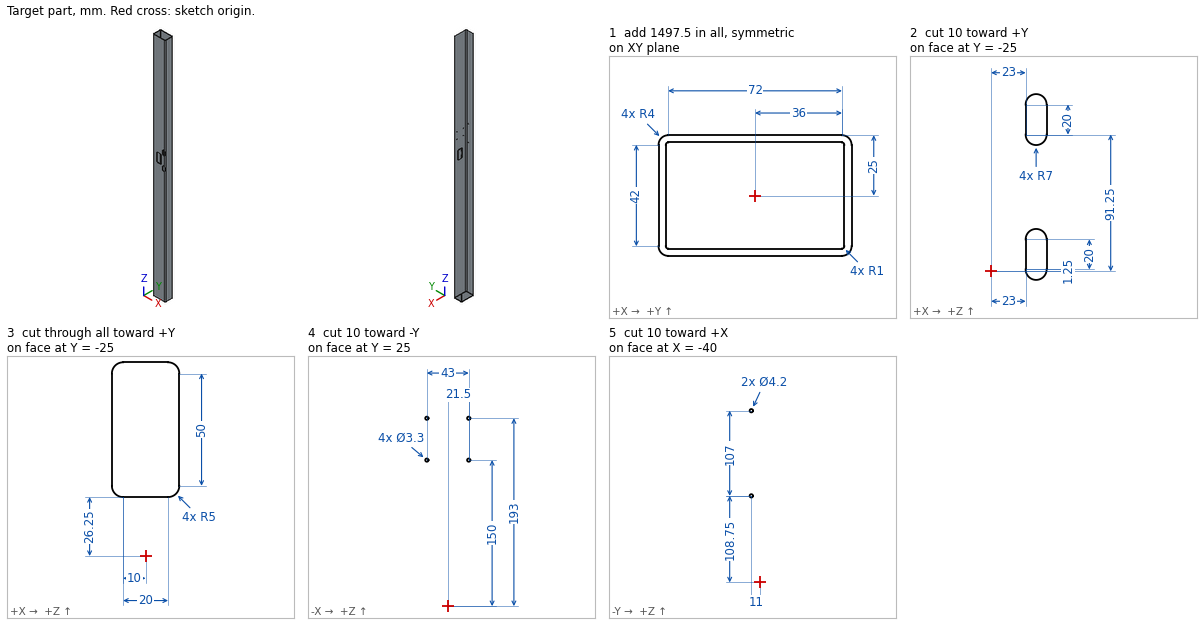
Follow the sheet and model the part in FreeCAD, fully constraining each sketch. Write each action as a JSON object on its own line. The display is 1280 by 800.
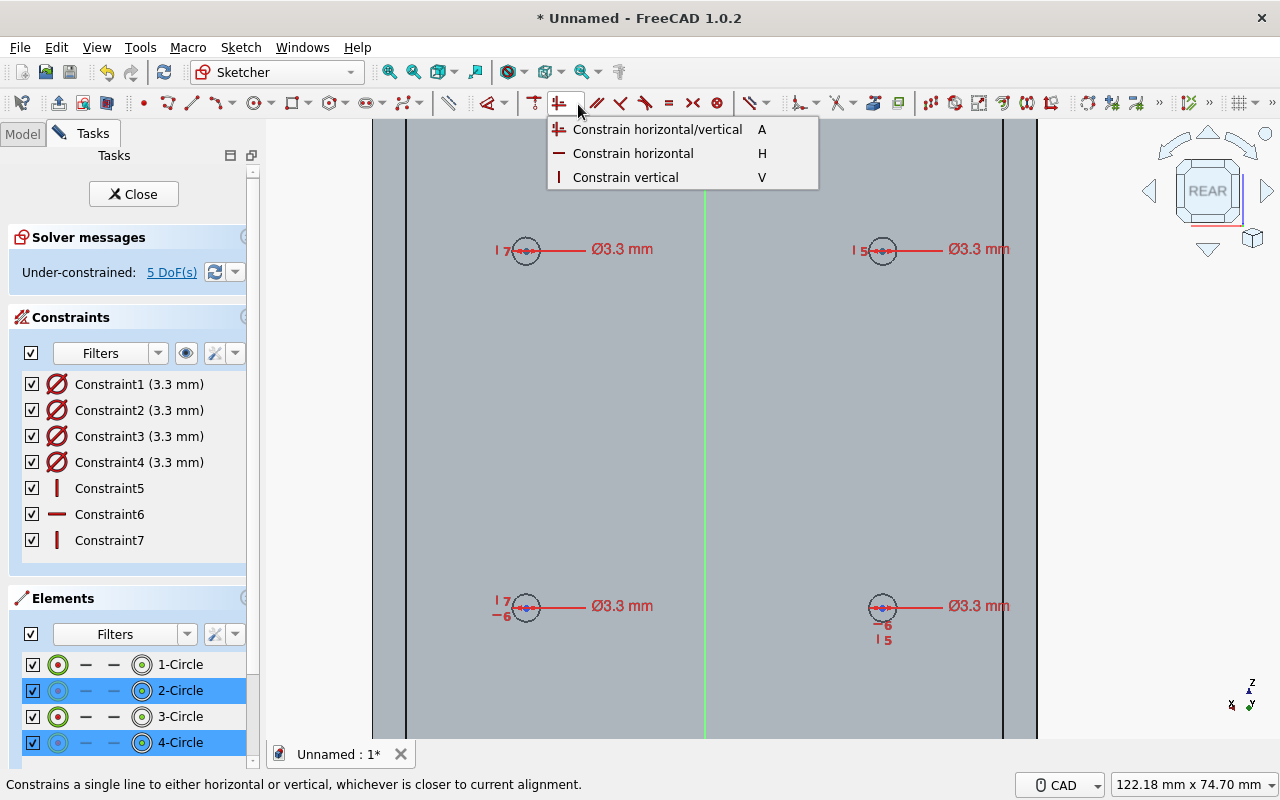
{"action": "left_click", "coordinate": [683, 153]}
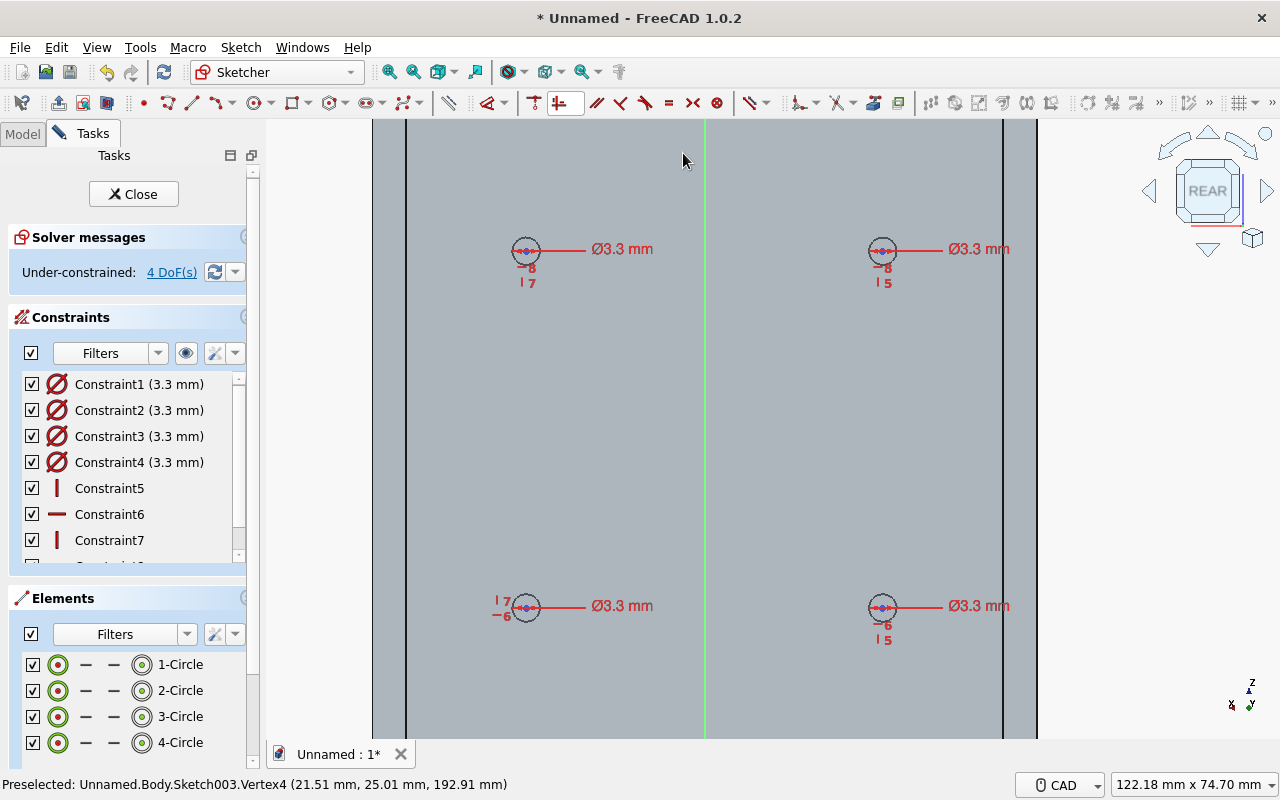
{"action": "left_click", "coordinate": [488, 104]}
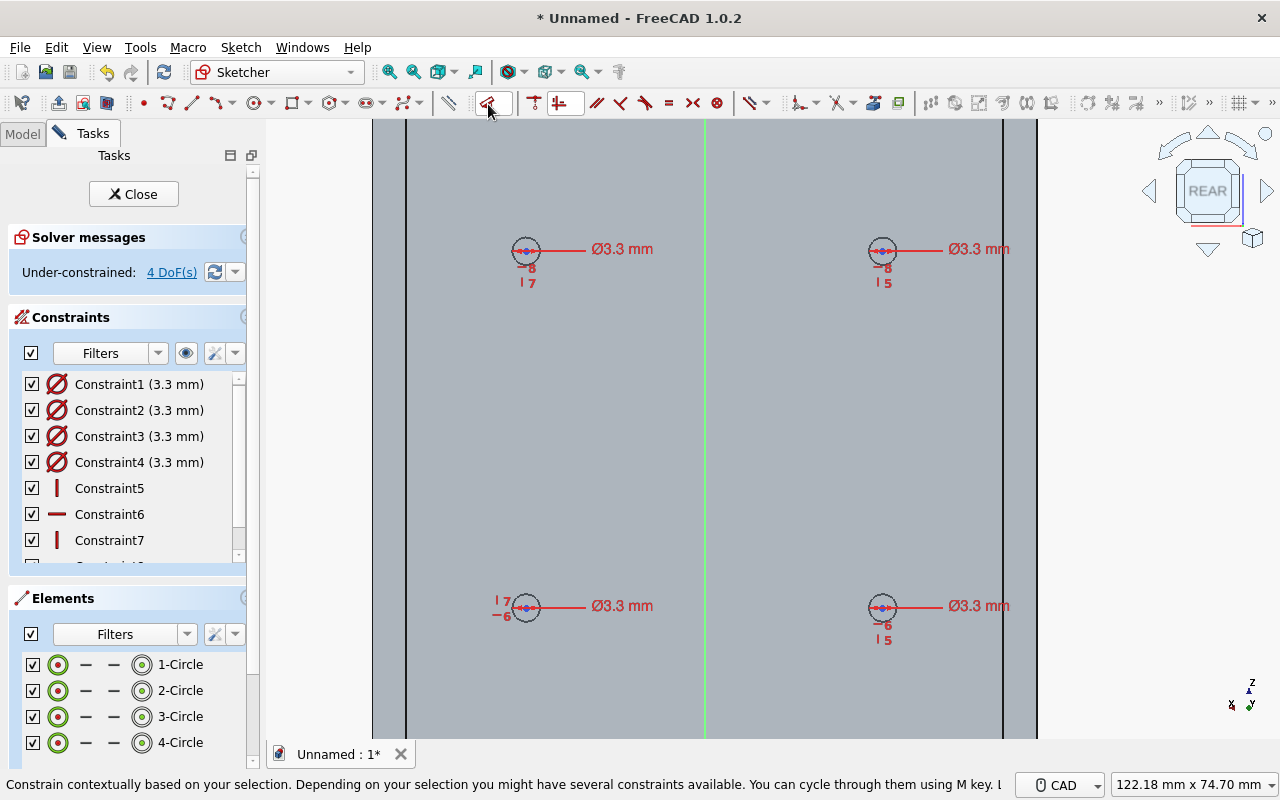
{"action": "left_click", "coordinate": [883, 608]}
{"action": "left_click", "coordinate": [917, 660]}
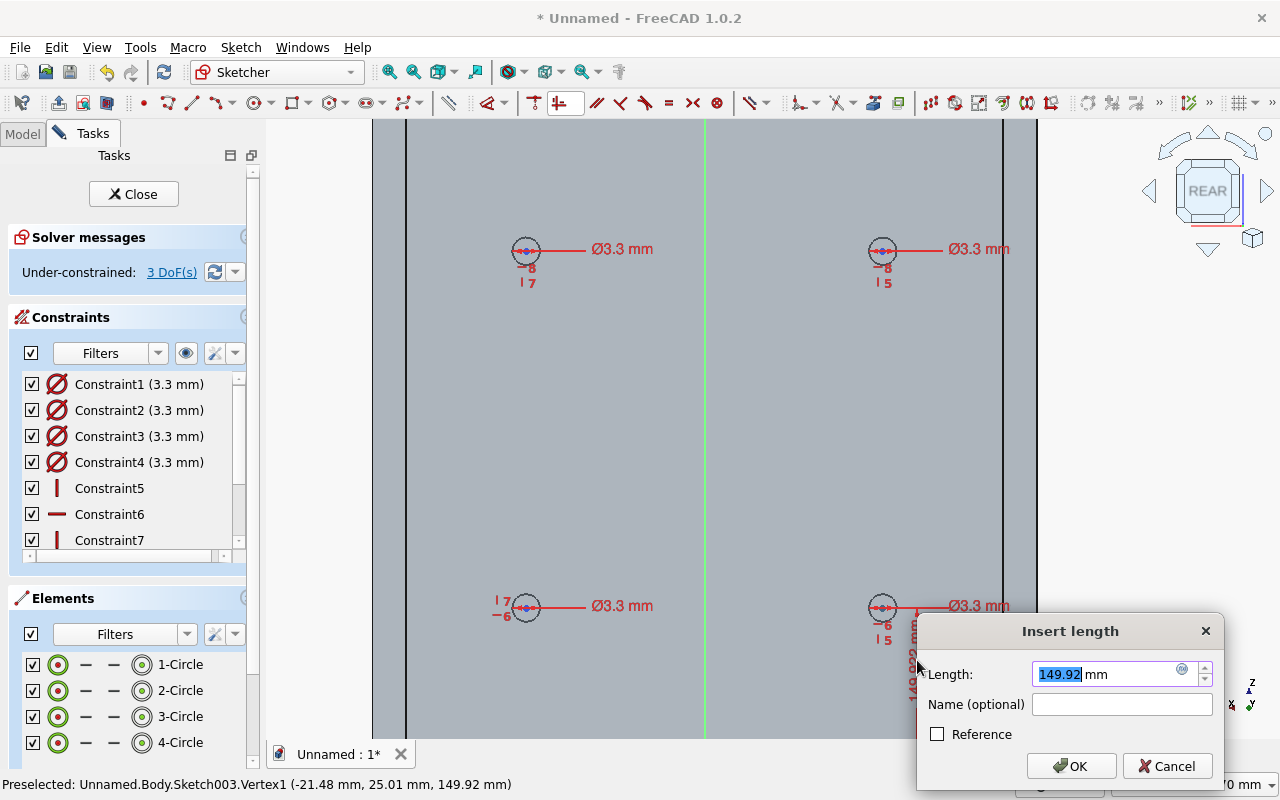
{"action": "type", "text": "150"}
{"action": "key", "text": "Return"}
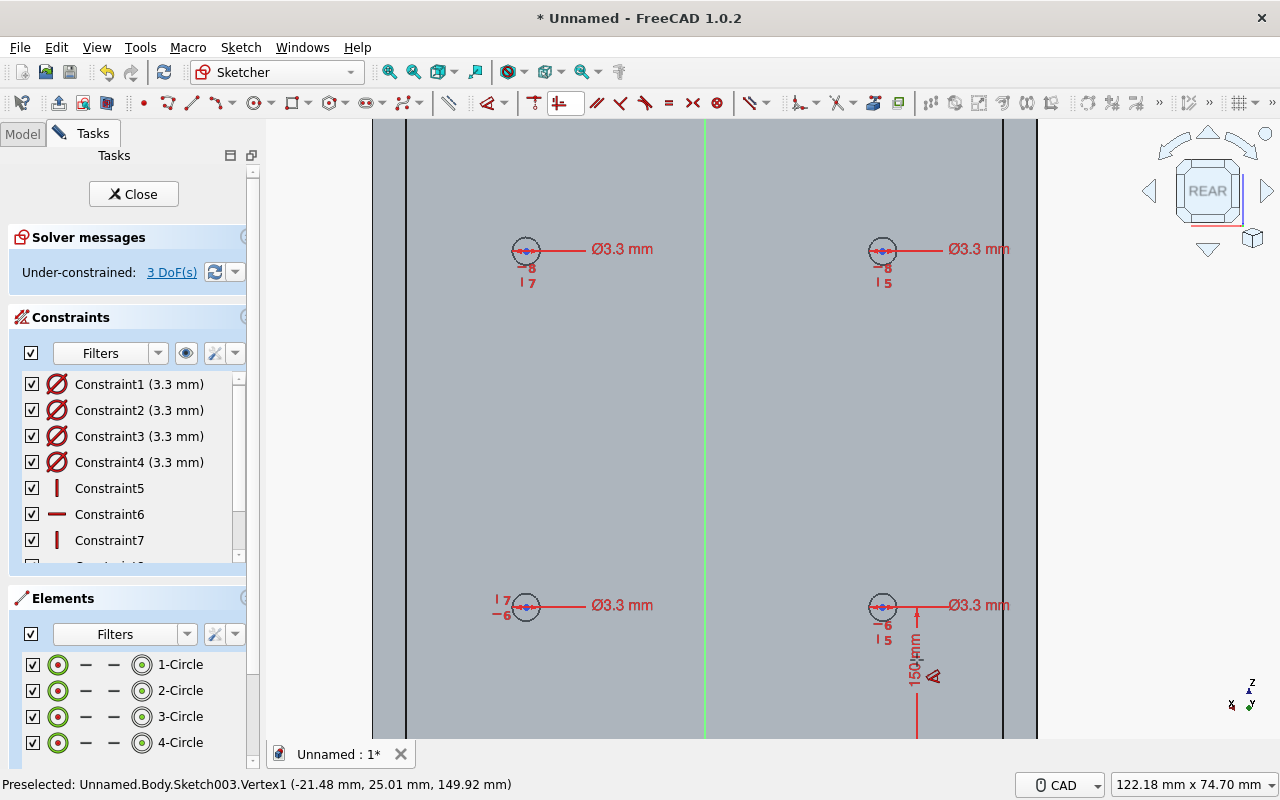
{"action": "left_click", "coordinate": [883, 251]}
{"action": "left_click", "coordinate": [917, 481]}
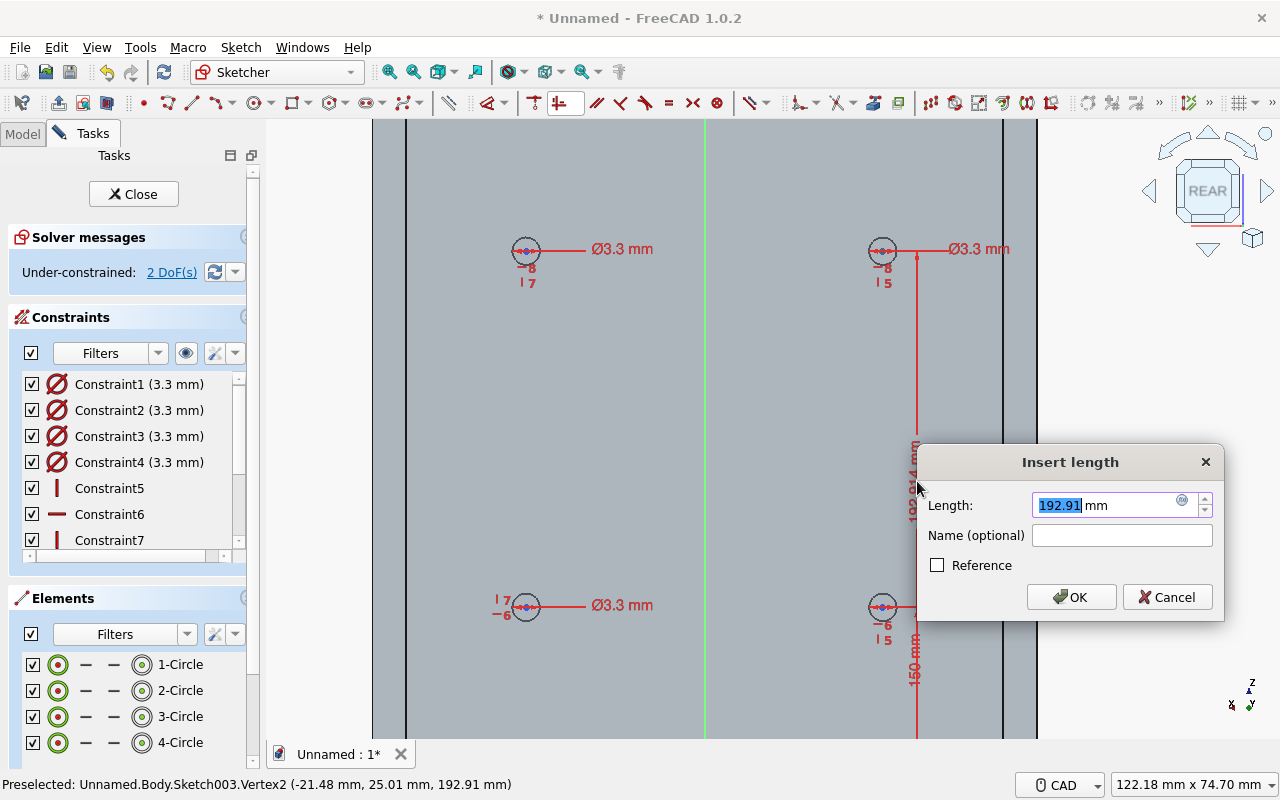
{"action": "type", "text": "193"}
{"action": "key", "text": "Return"}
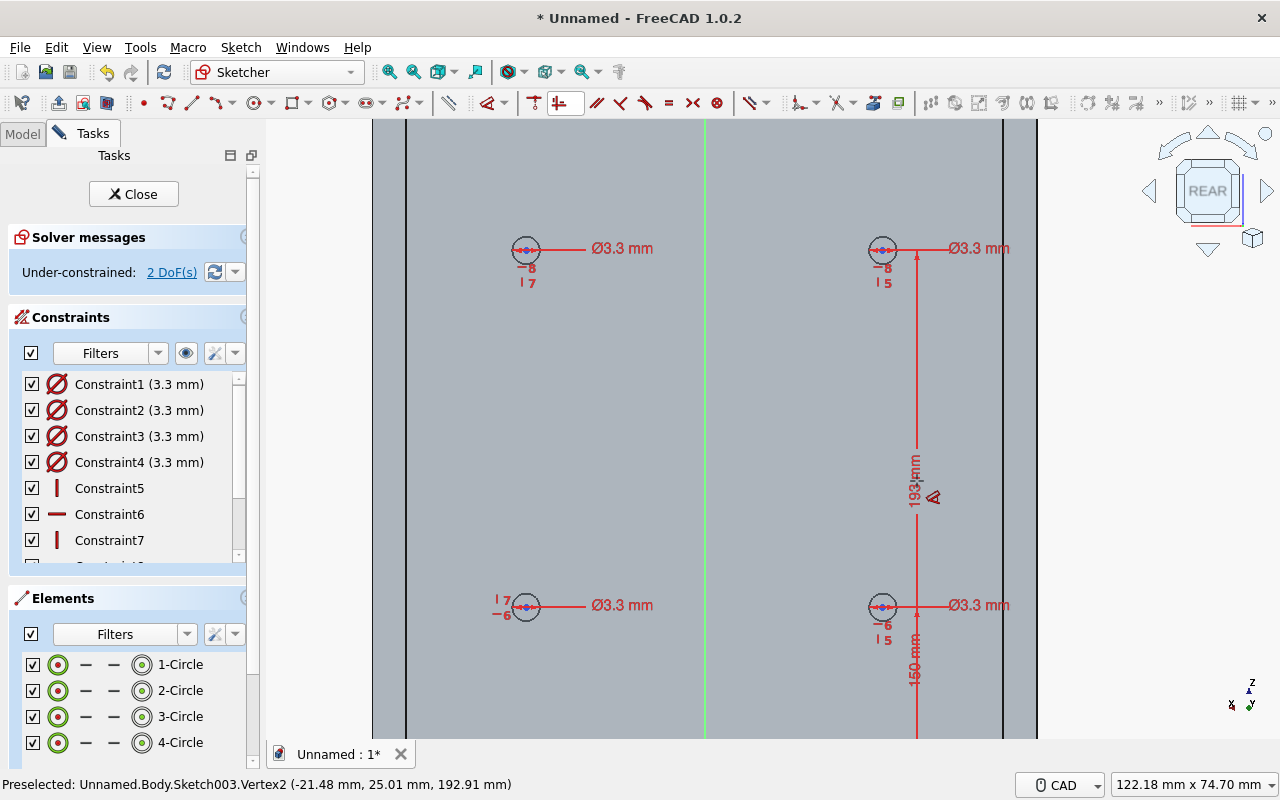
{"action": "left_click", "coordinate": [883, 607]}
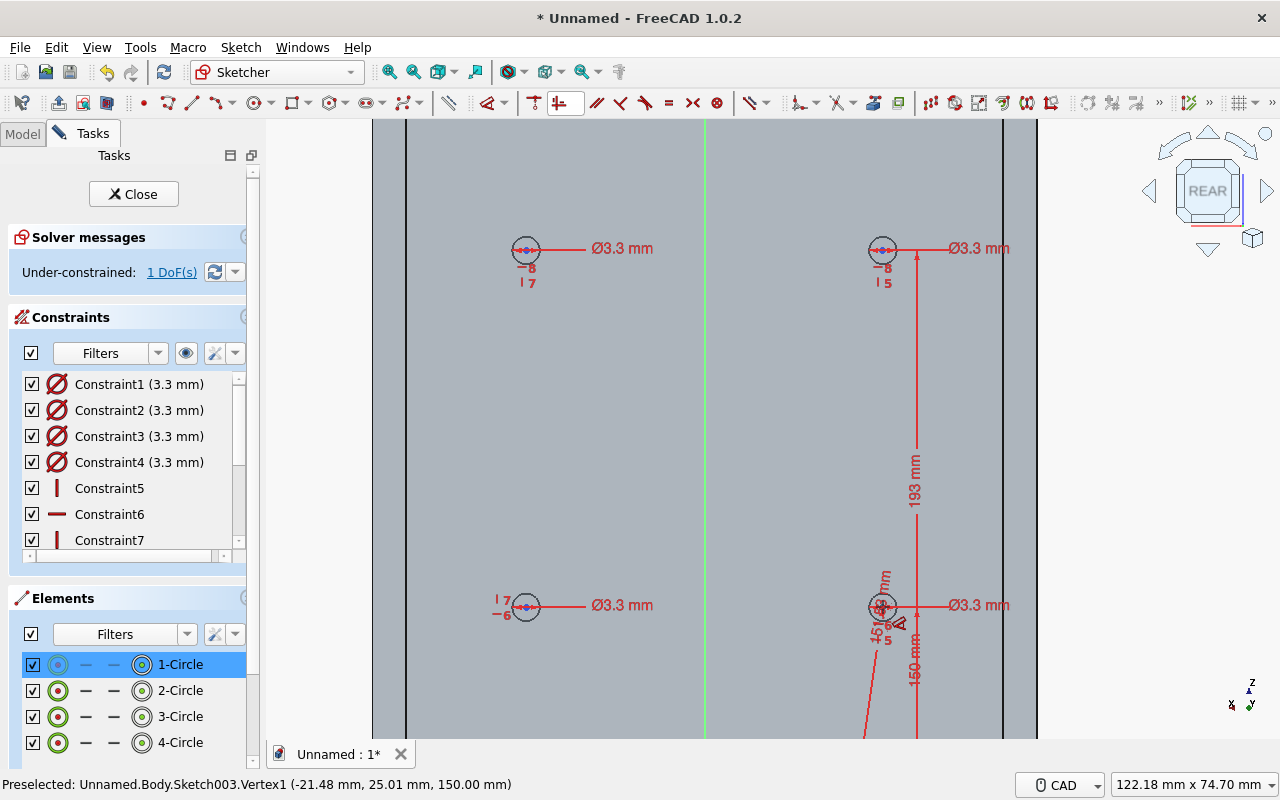
{"action": "left_click", "coordinate": [526, 607]}
{"action": "left_click", "coordinate": [622, 641]}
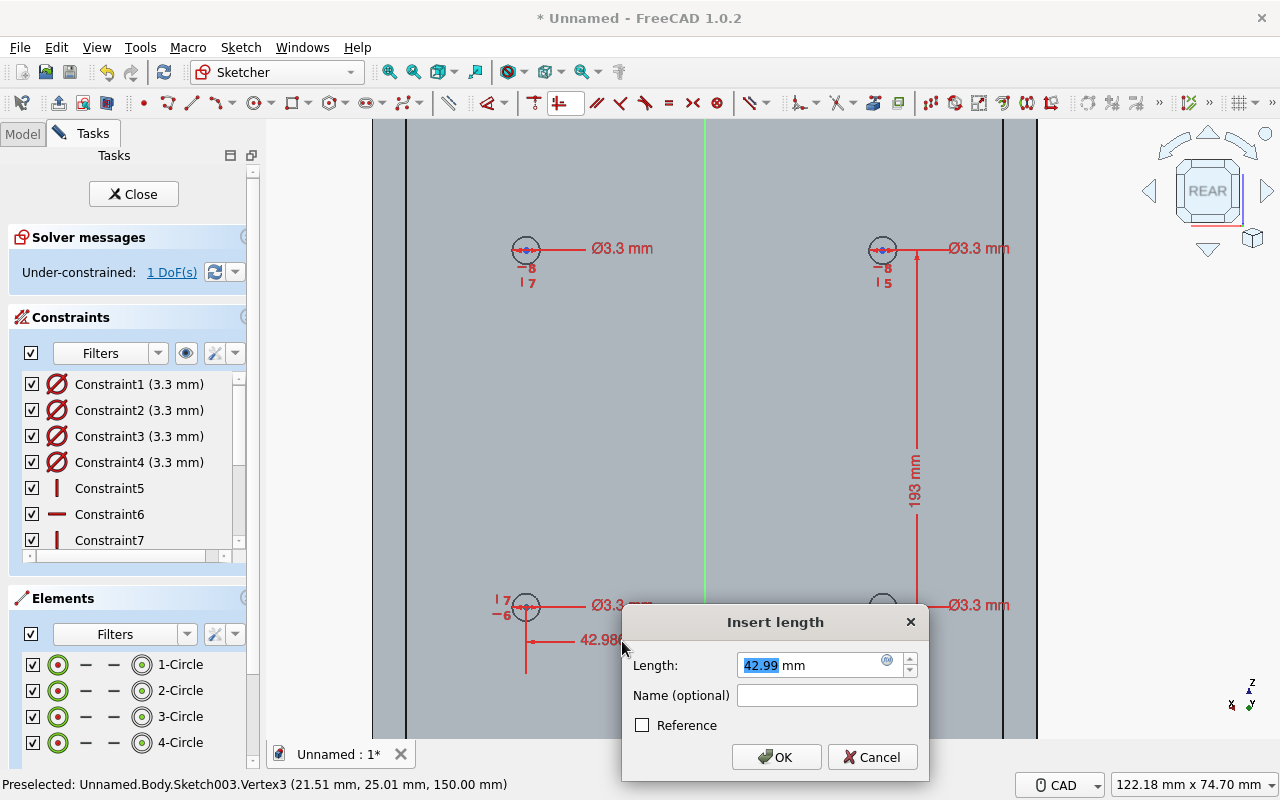
{"action": "type", "text": "43"}
{"action": "key", "text": "Return"}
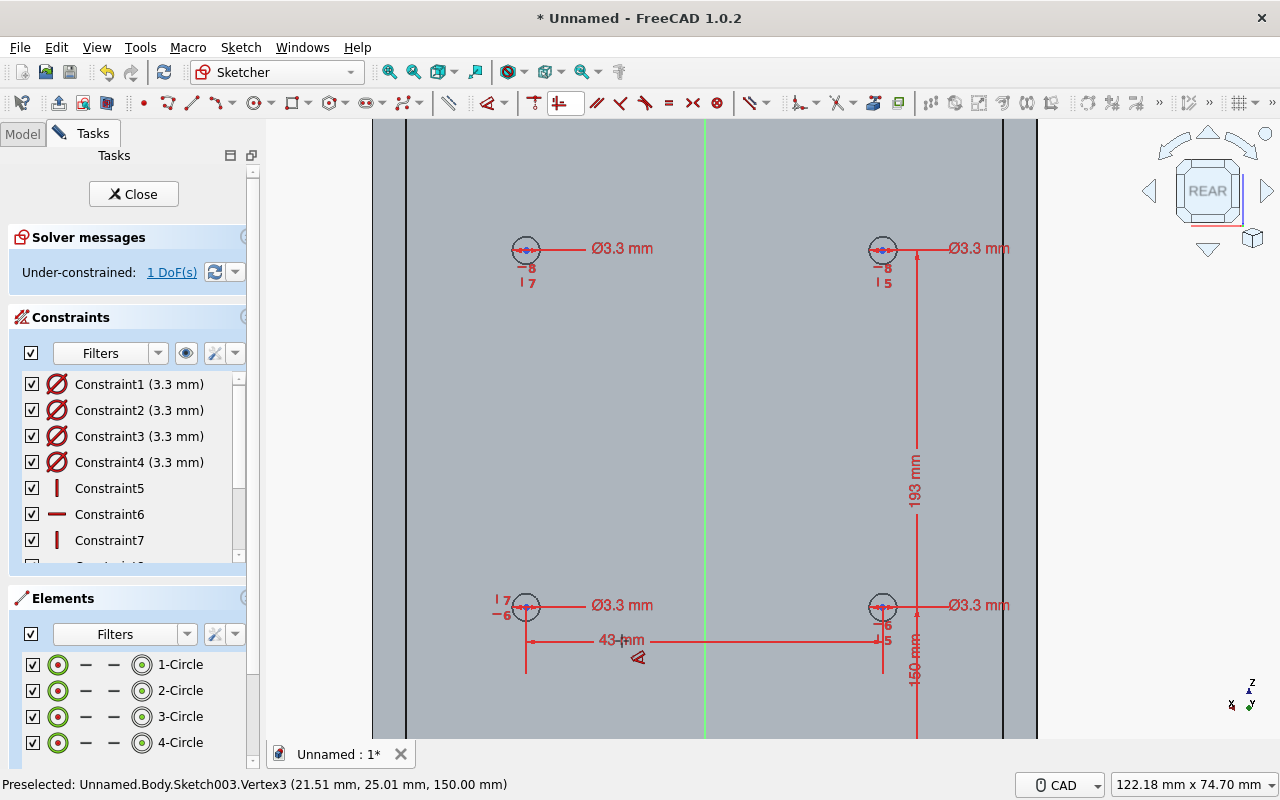
{"action": "left_click", "coordinate": [883, 607]}
{"action": "left_click", "coordinate": [794, 573]}